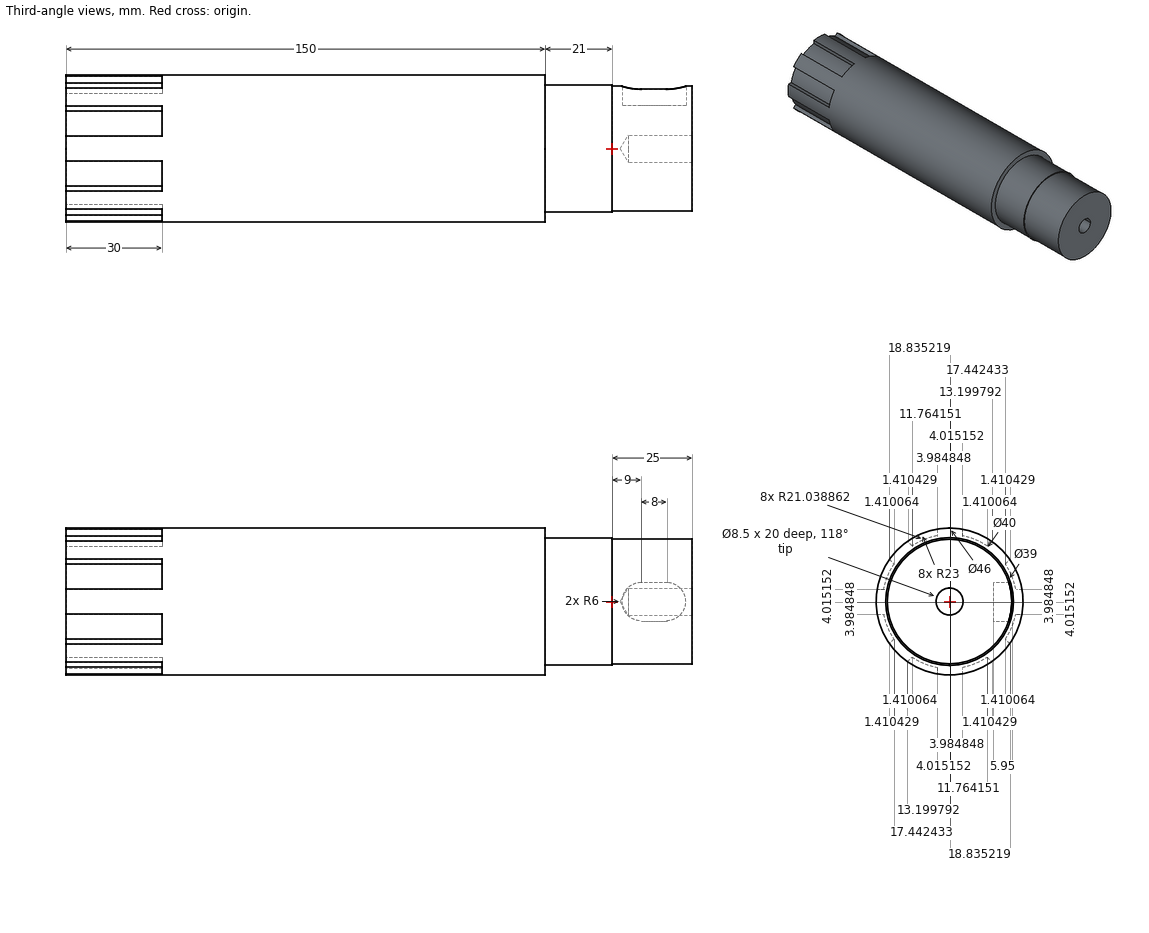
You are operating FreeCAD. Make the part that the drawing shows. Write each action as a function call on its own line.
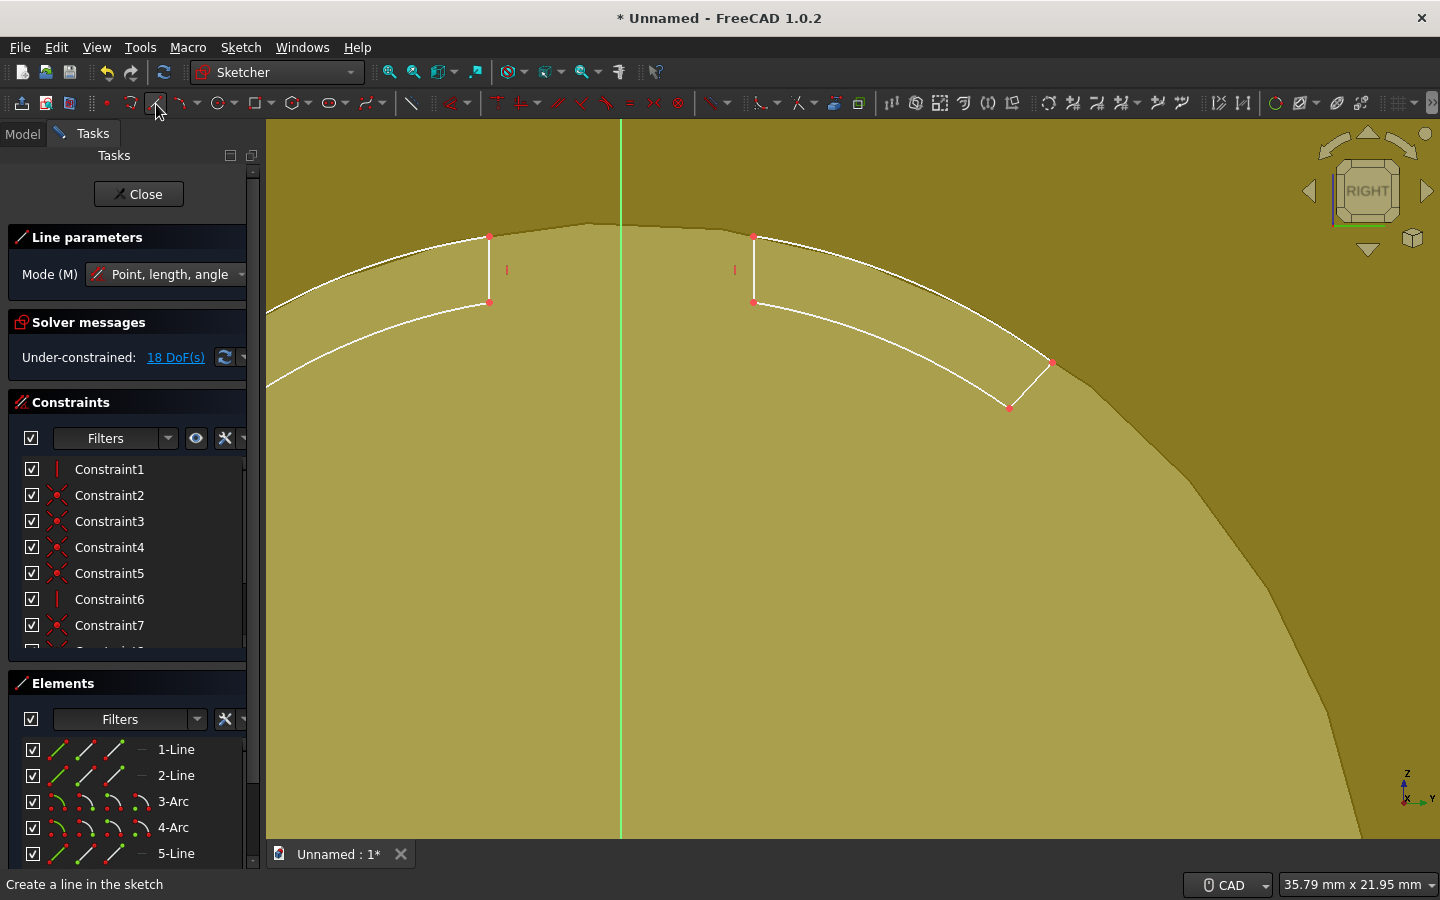
scroll(855, 264, down, 6)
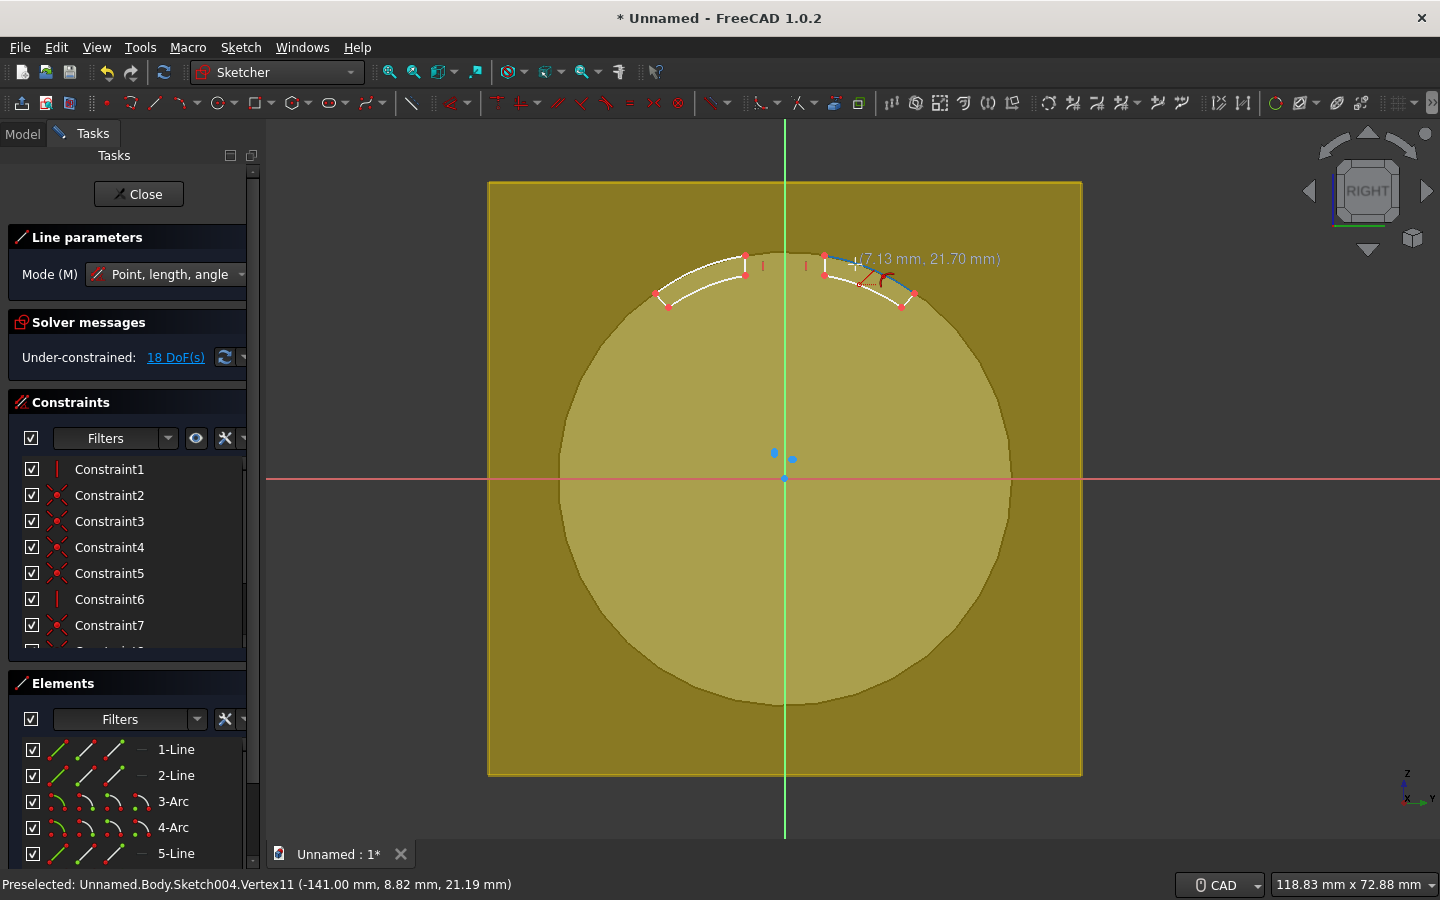
click(745, 683)
click(745, 703)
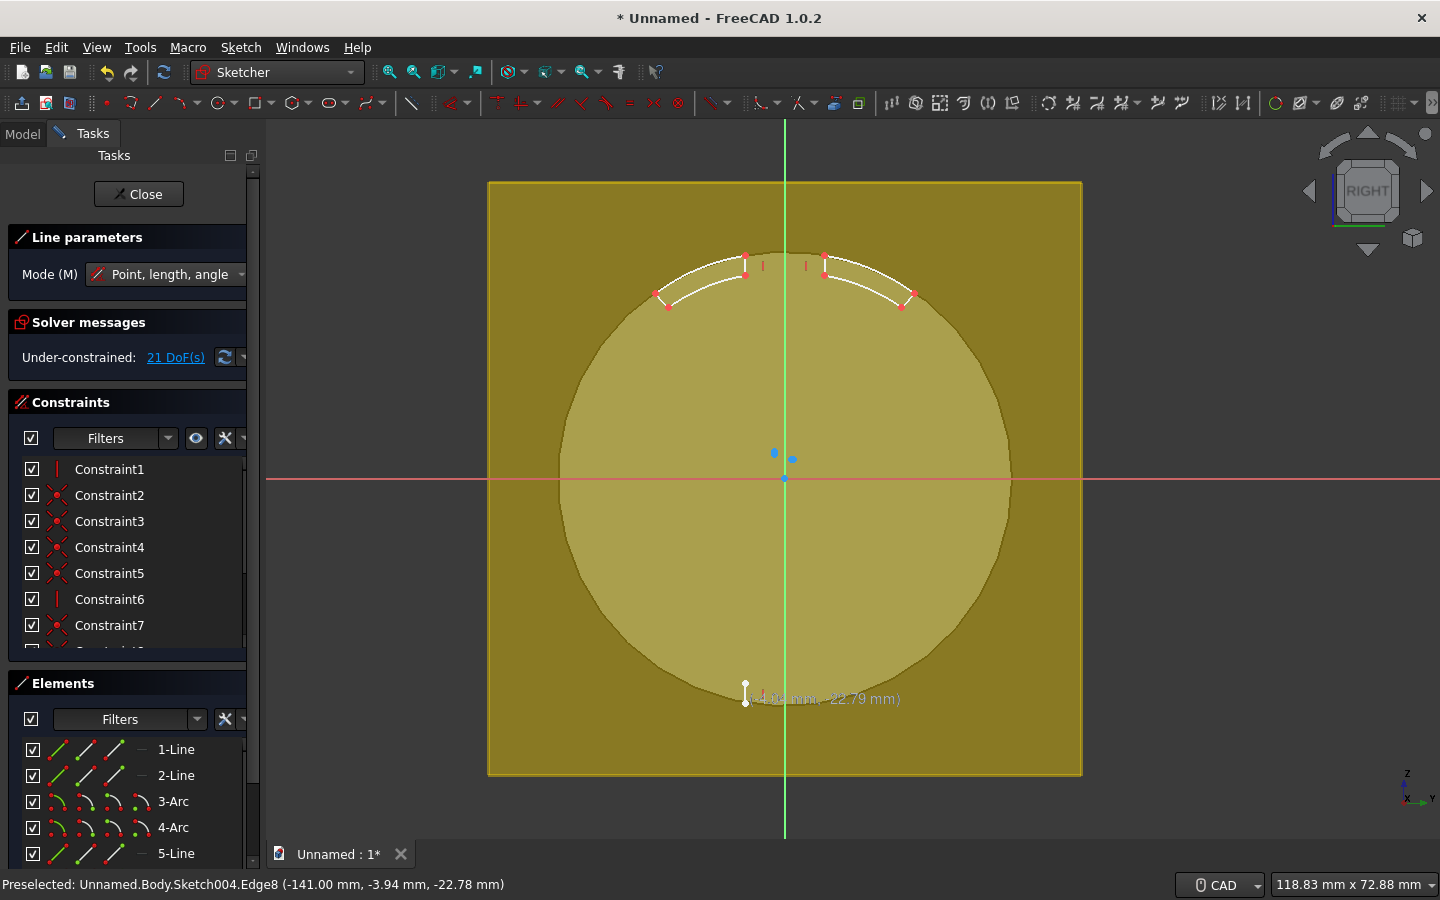
click(654, 665)
click(668, 651)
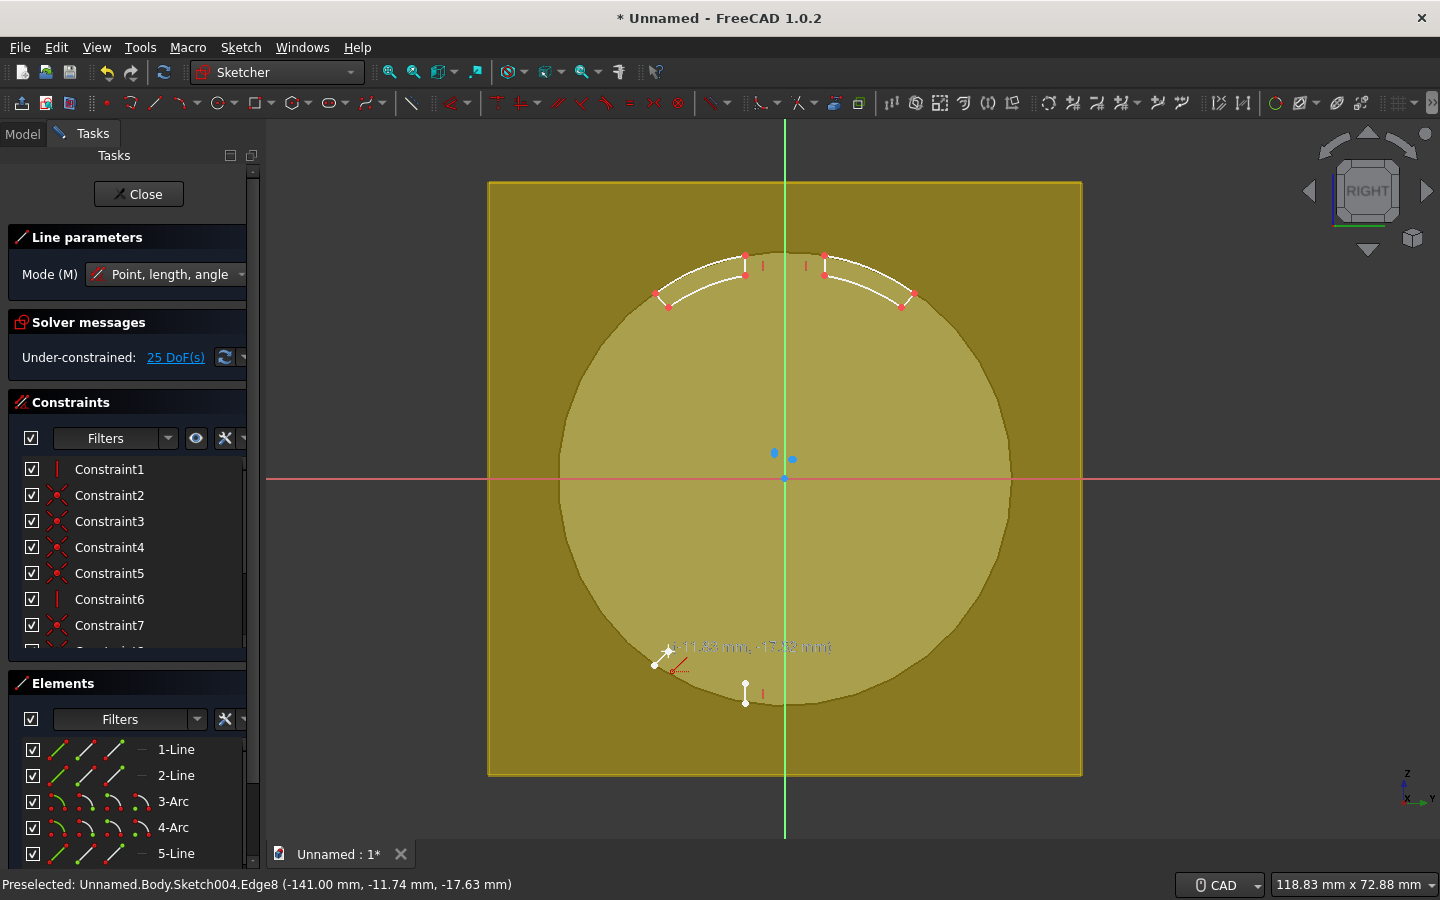
click(180, 104)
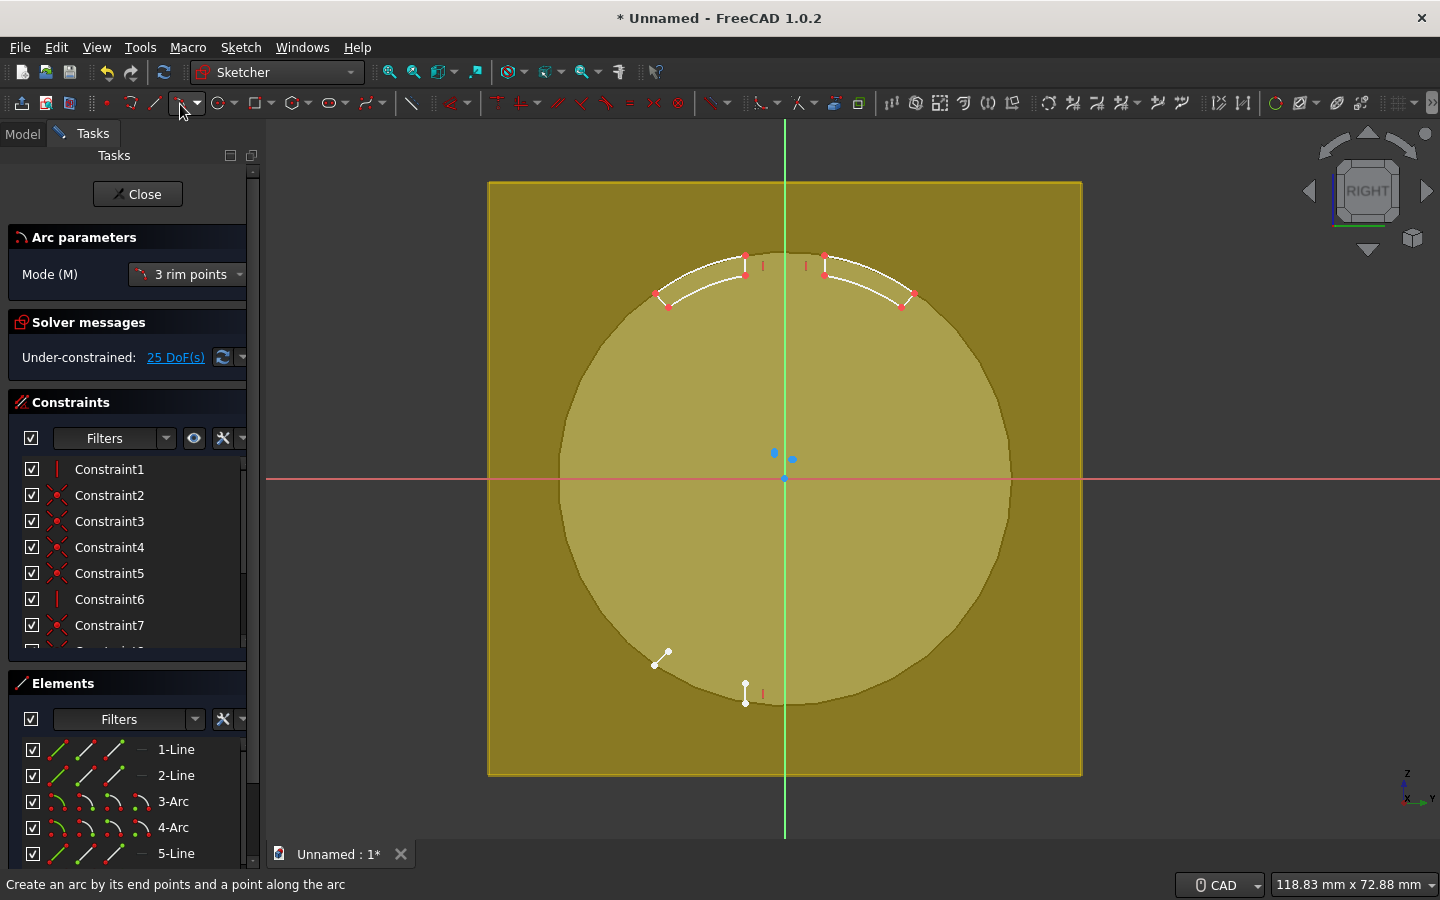
scroll(745, 703, up, 3)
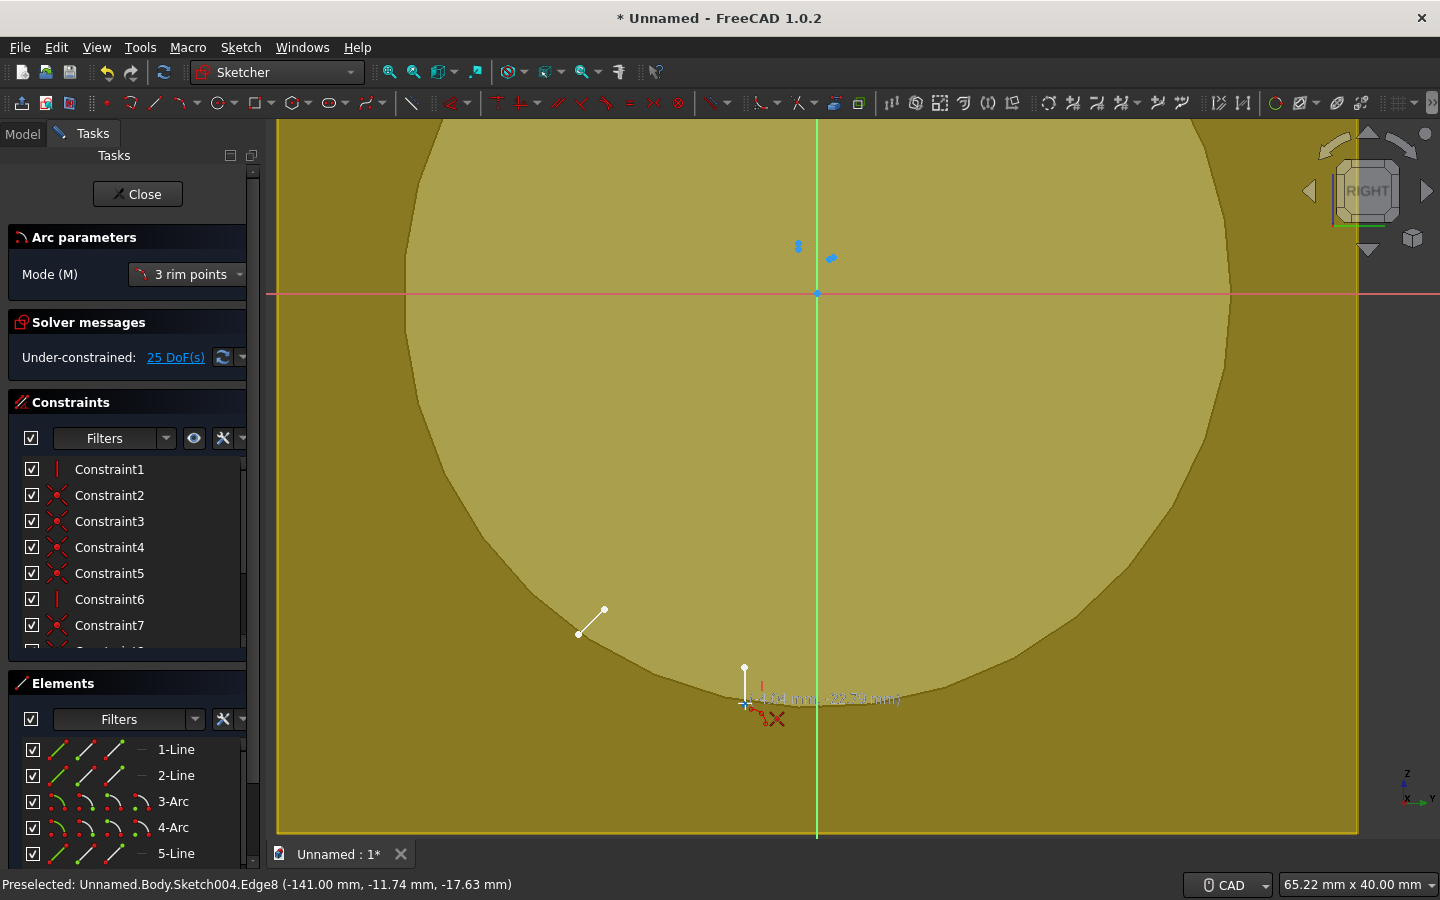
click(745, 704)
click(579, 635)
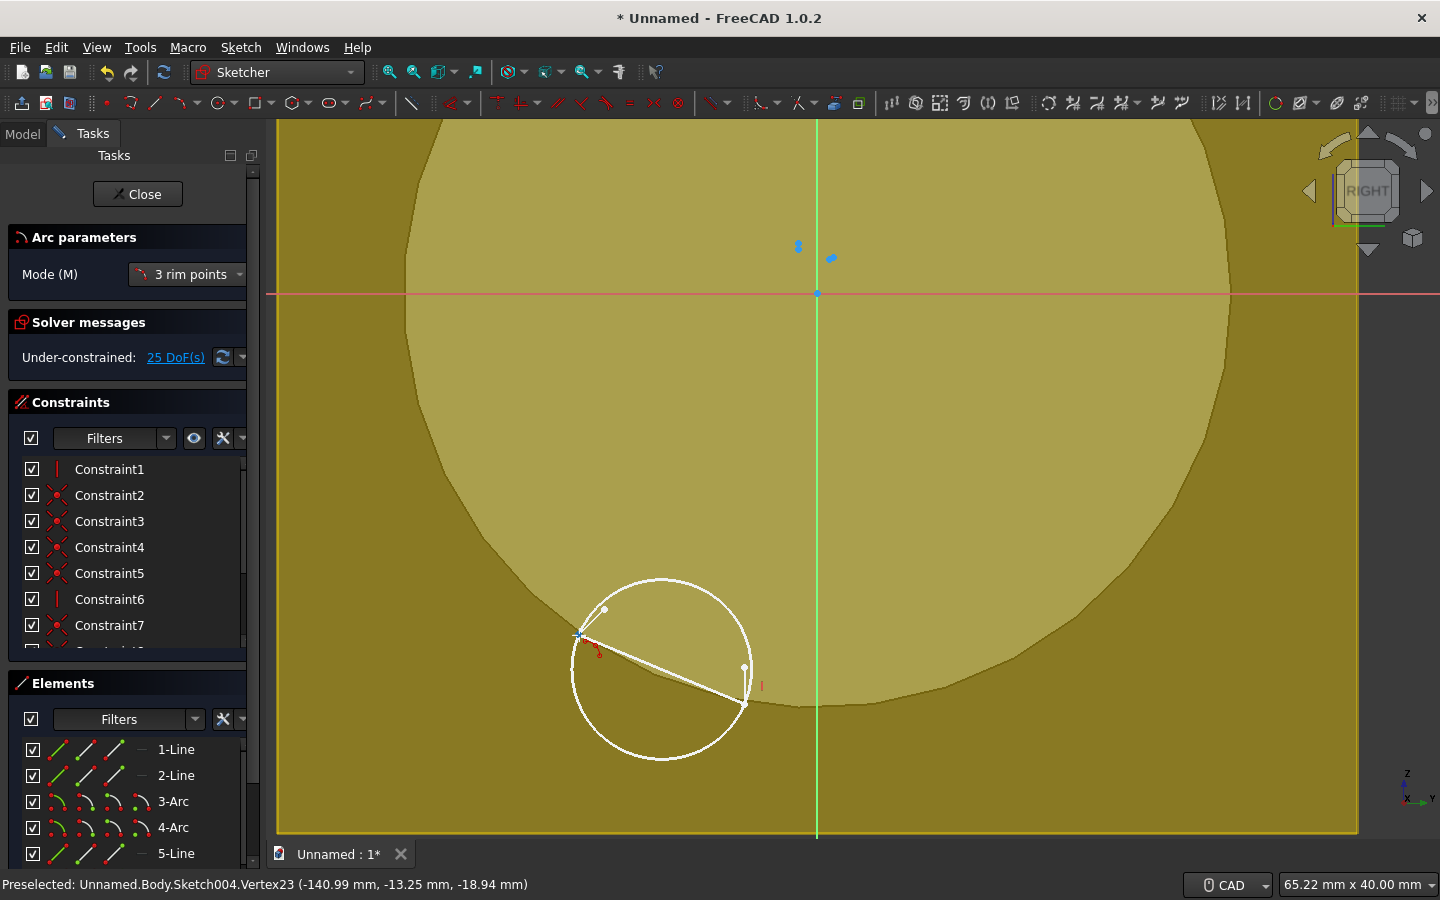
scroll(659, 676, up, 3)